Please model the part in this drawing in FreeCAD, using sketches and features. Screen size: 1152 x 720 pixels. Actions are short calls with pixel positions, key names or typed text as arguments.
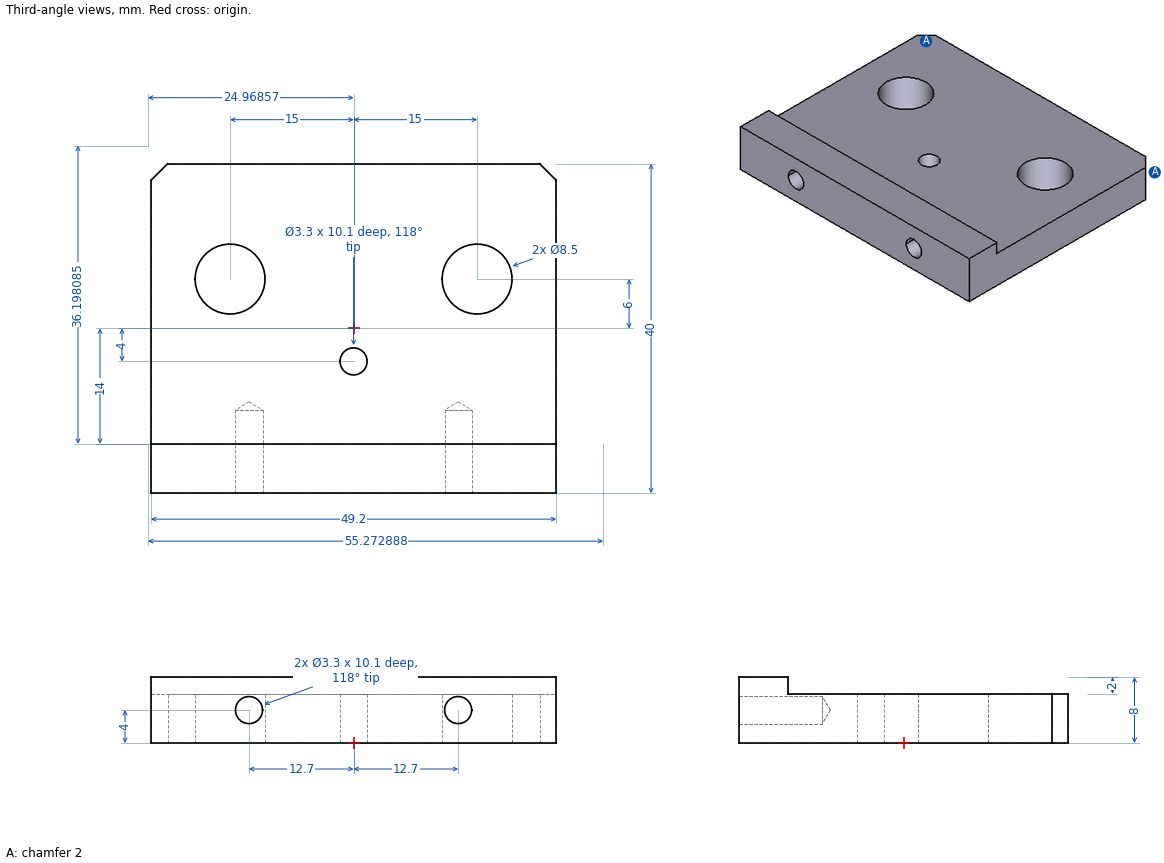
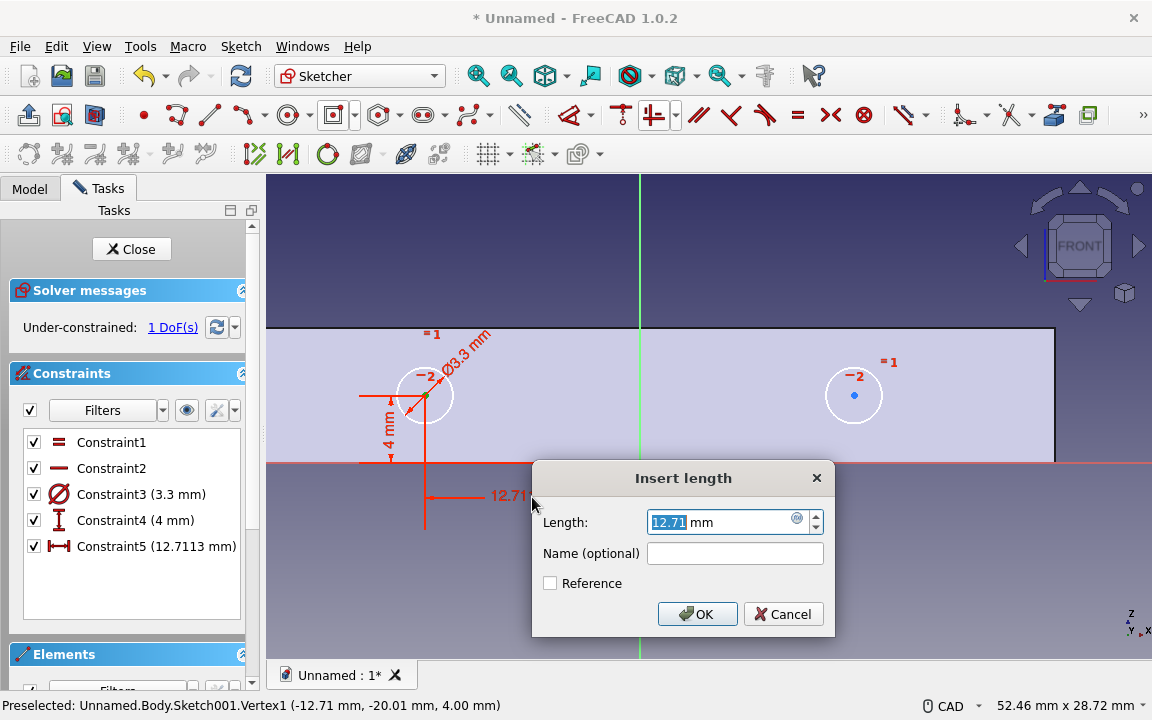
text(12.7)
key(Return)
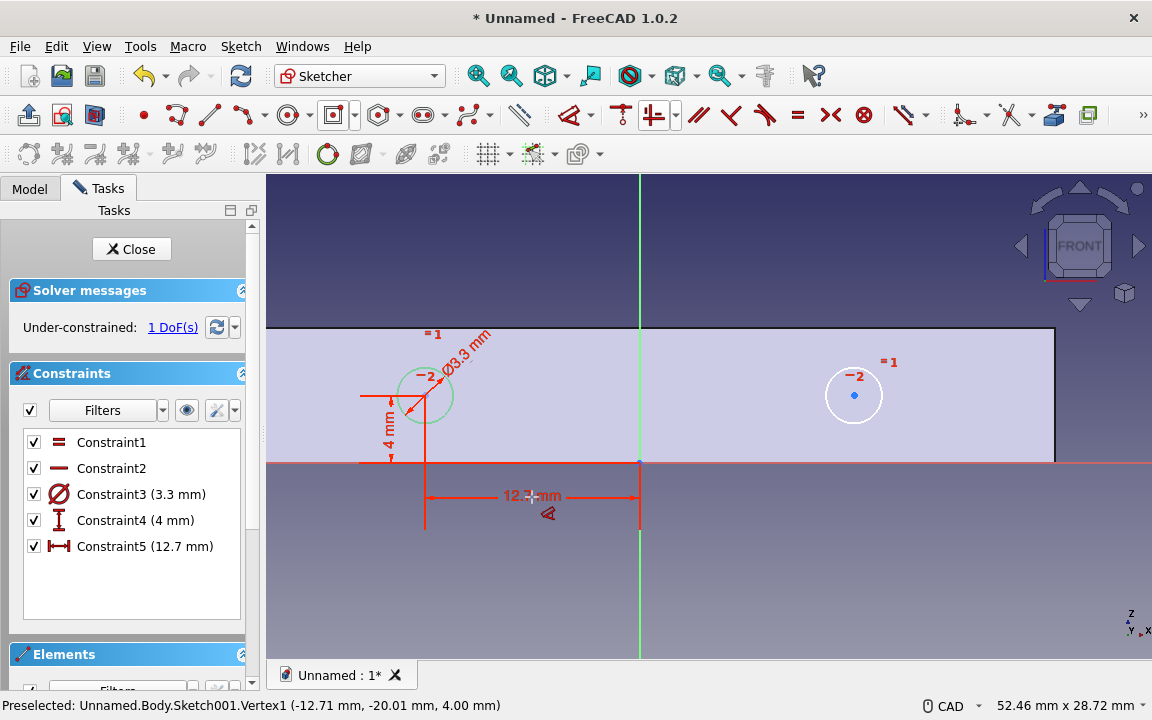
click(854, 396)
click(747, 497)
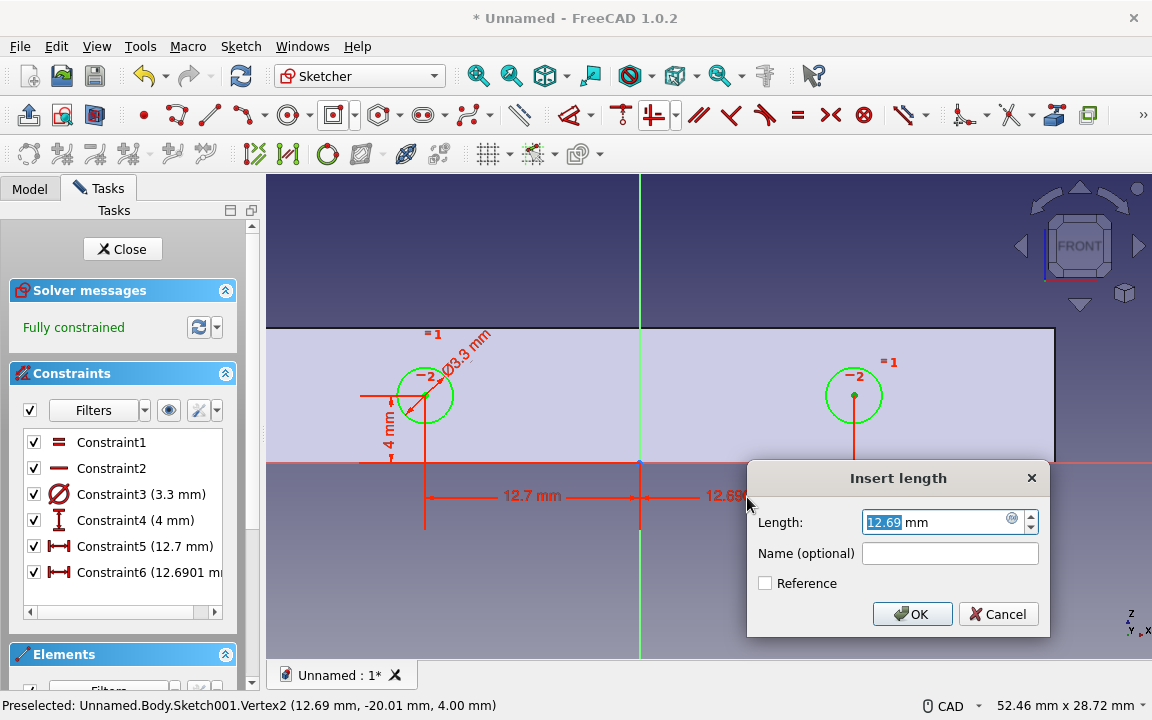
text(12.7)
key(Return)
key(Escape)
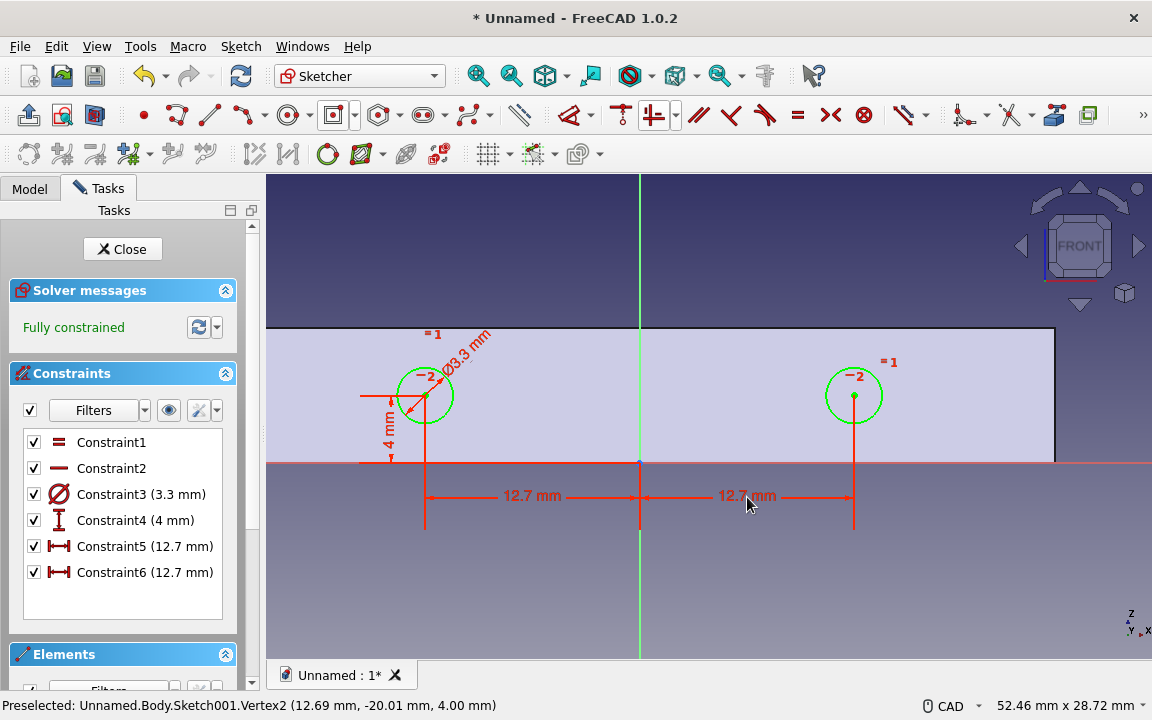
click(123, 249)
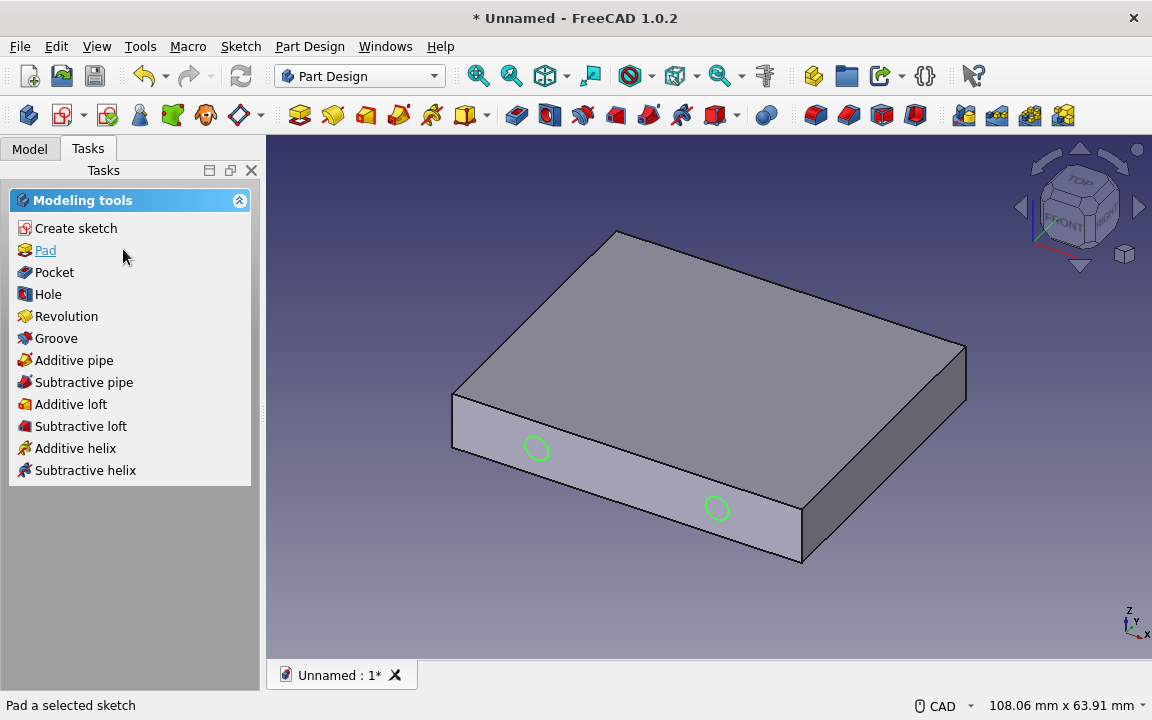
click(550, 116)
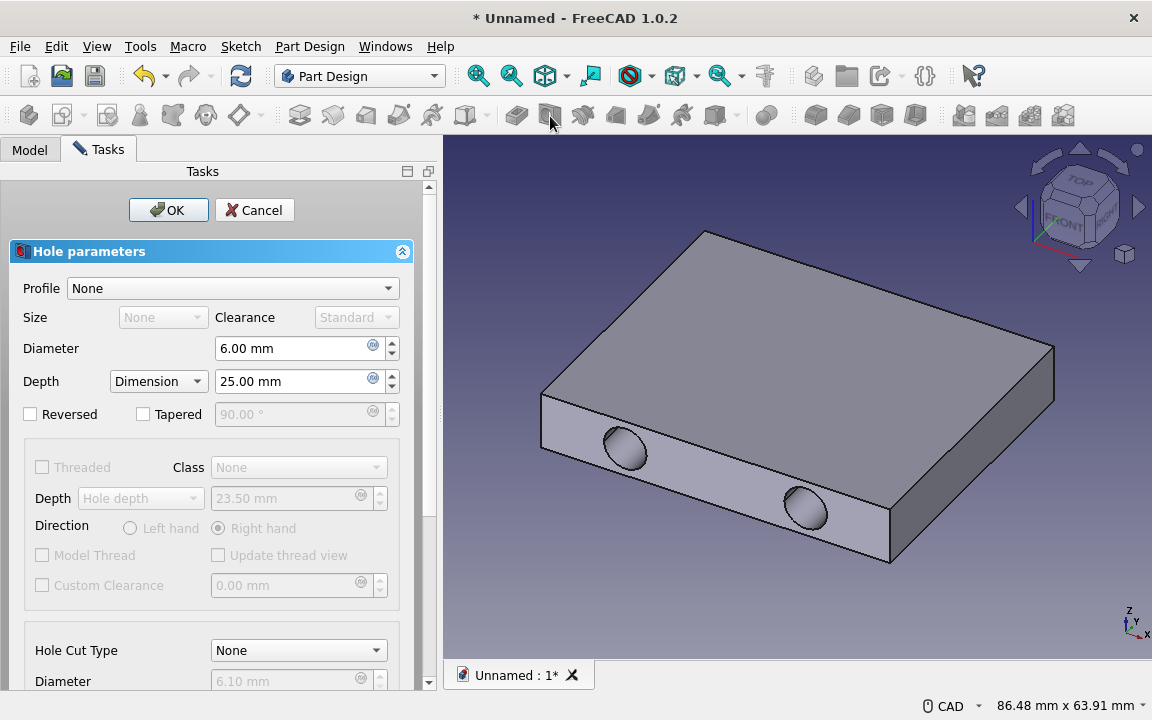
triple_click(300, 348)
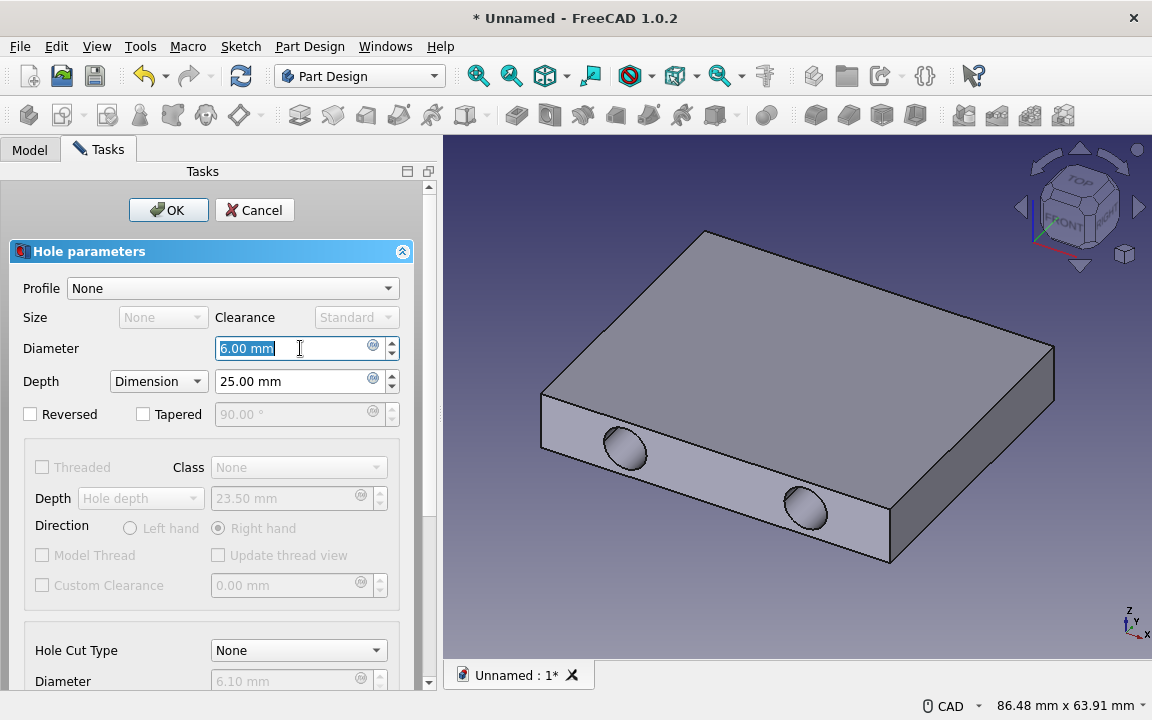
text(3.3)
key(Tab)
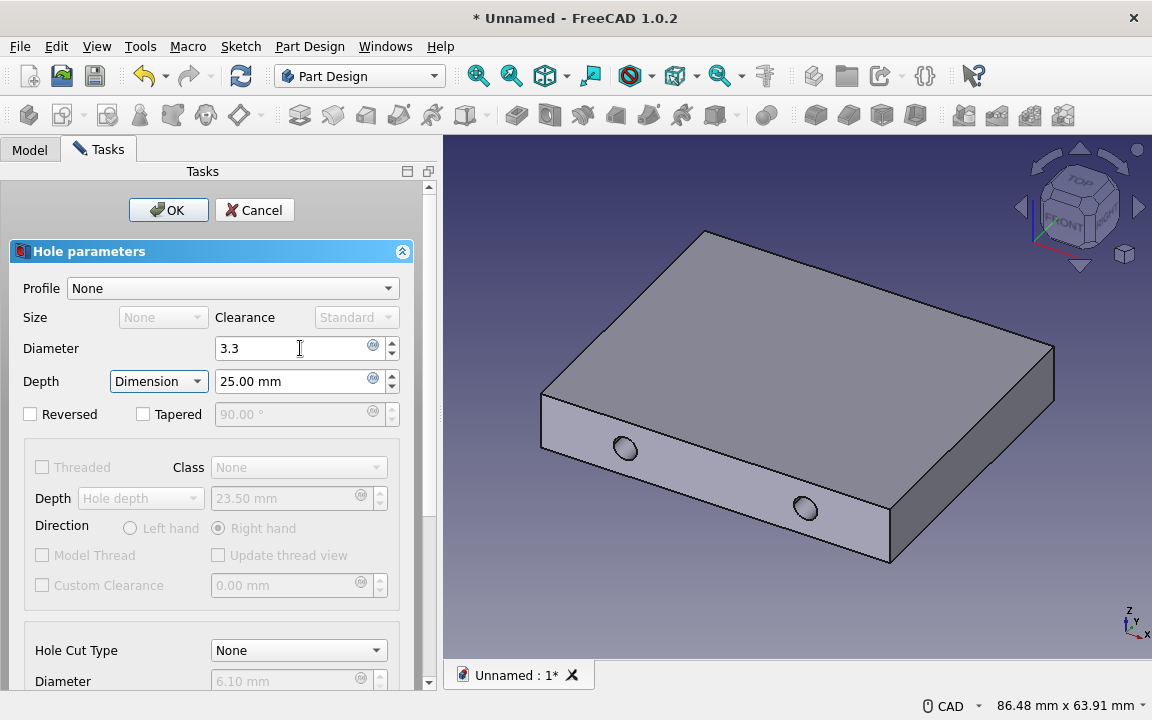
triple_click(300, 382)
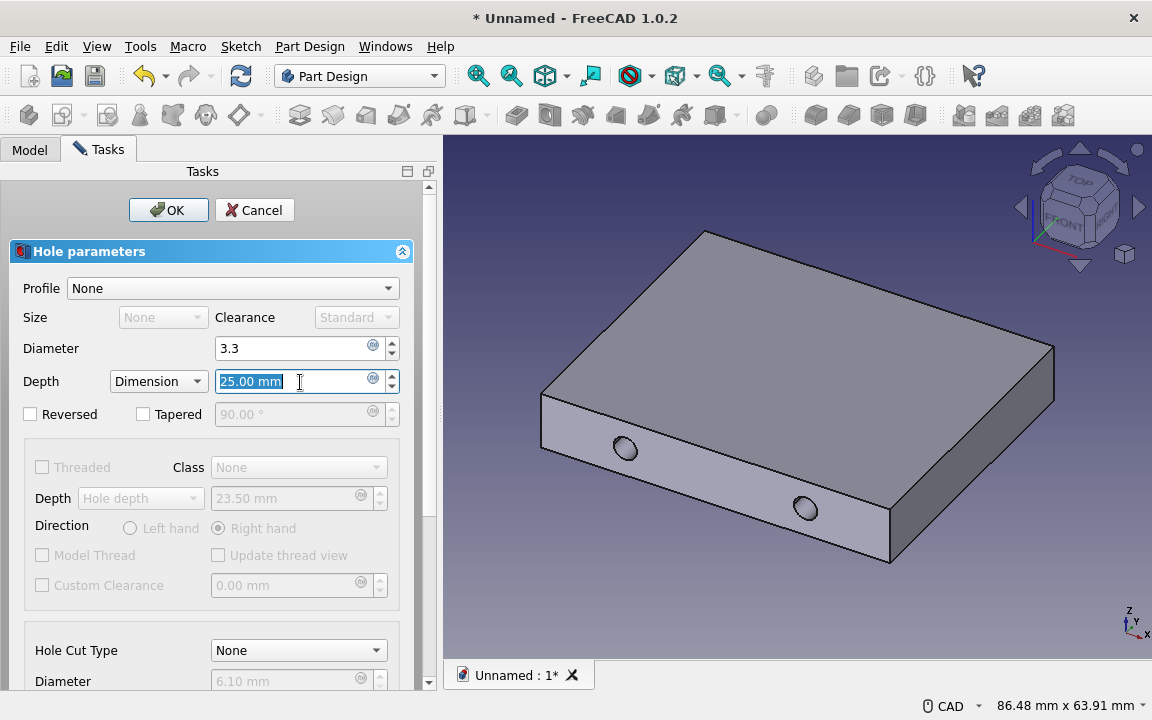
text(10.1)
key(Tab)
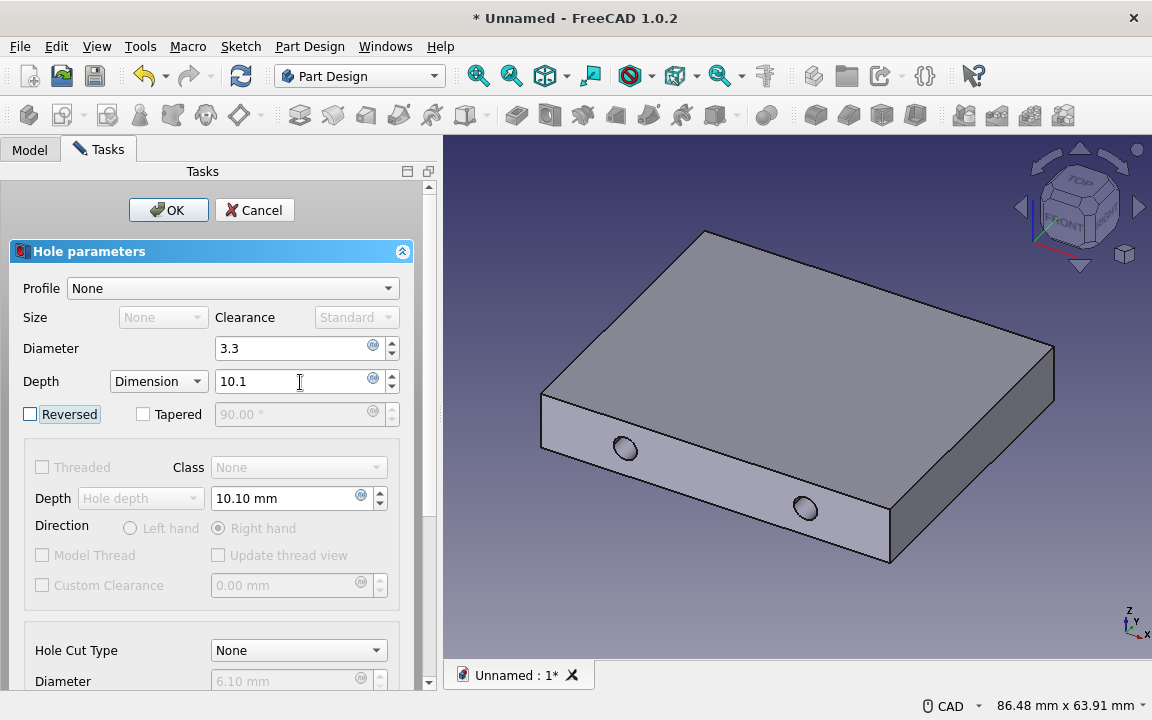
click(169, 210)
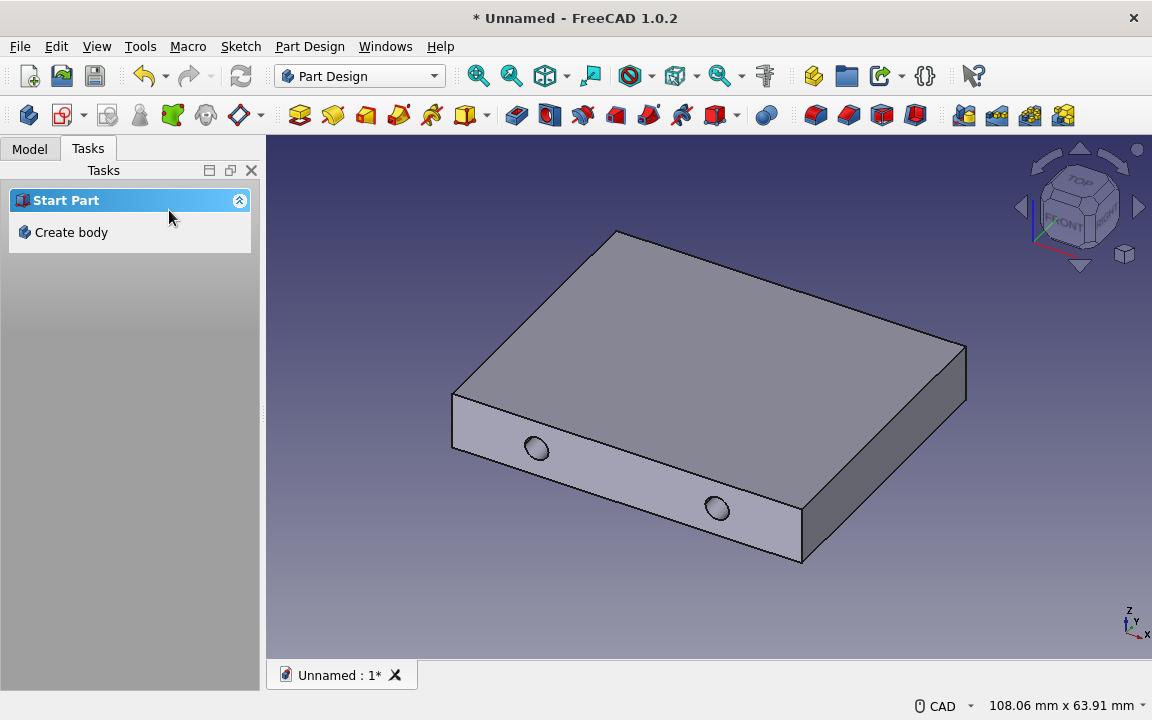
key(0)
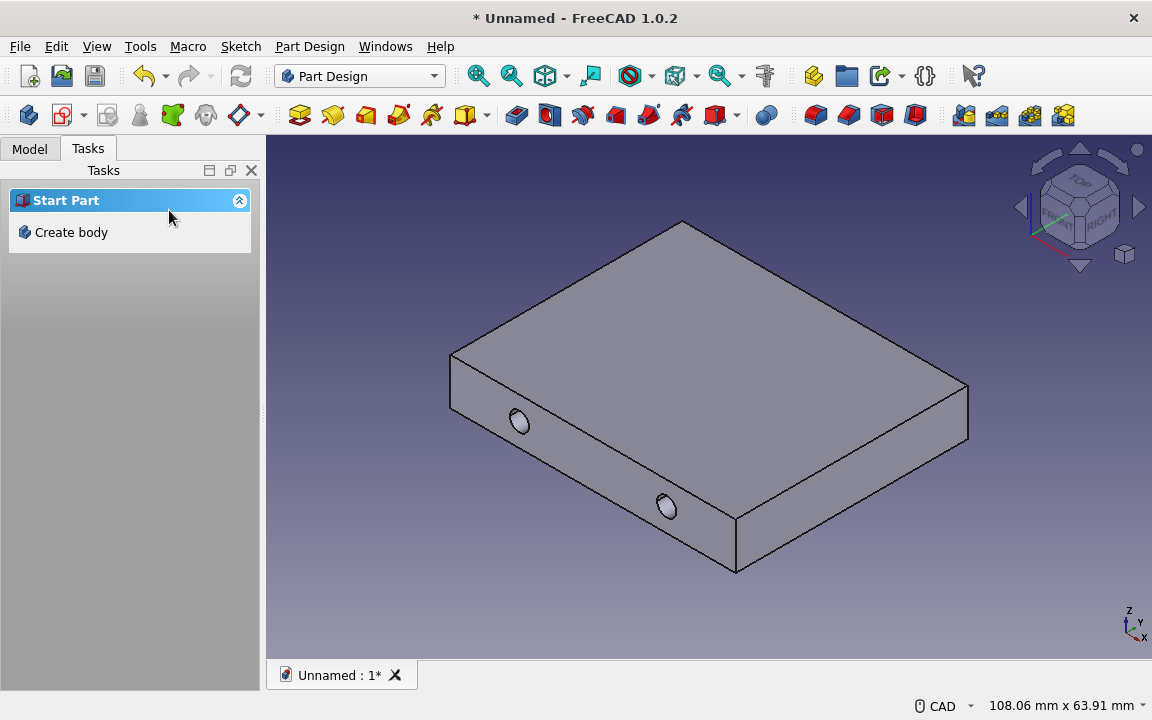
key(2)